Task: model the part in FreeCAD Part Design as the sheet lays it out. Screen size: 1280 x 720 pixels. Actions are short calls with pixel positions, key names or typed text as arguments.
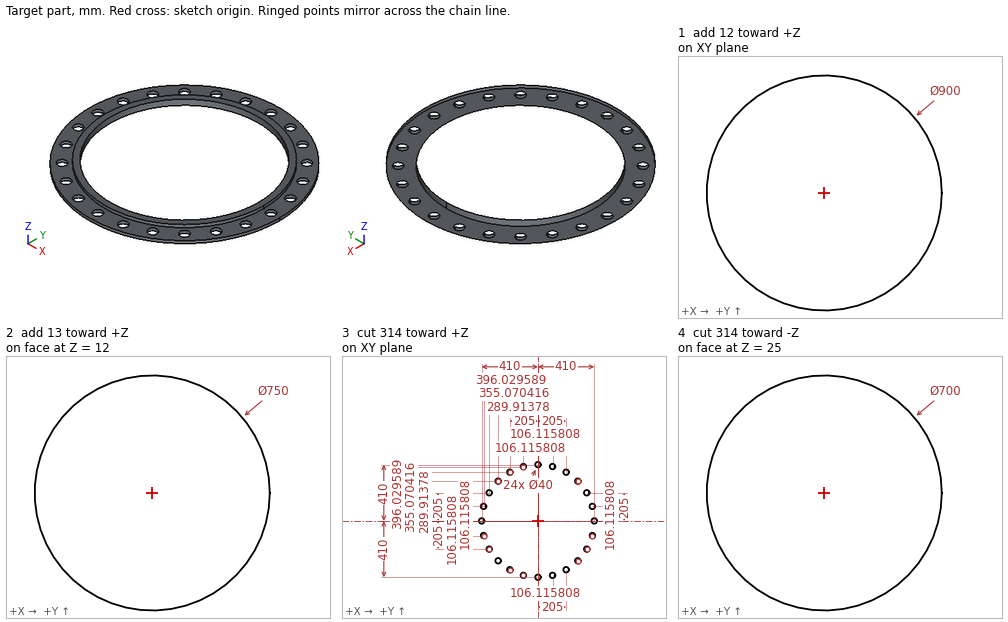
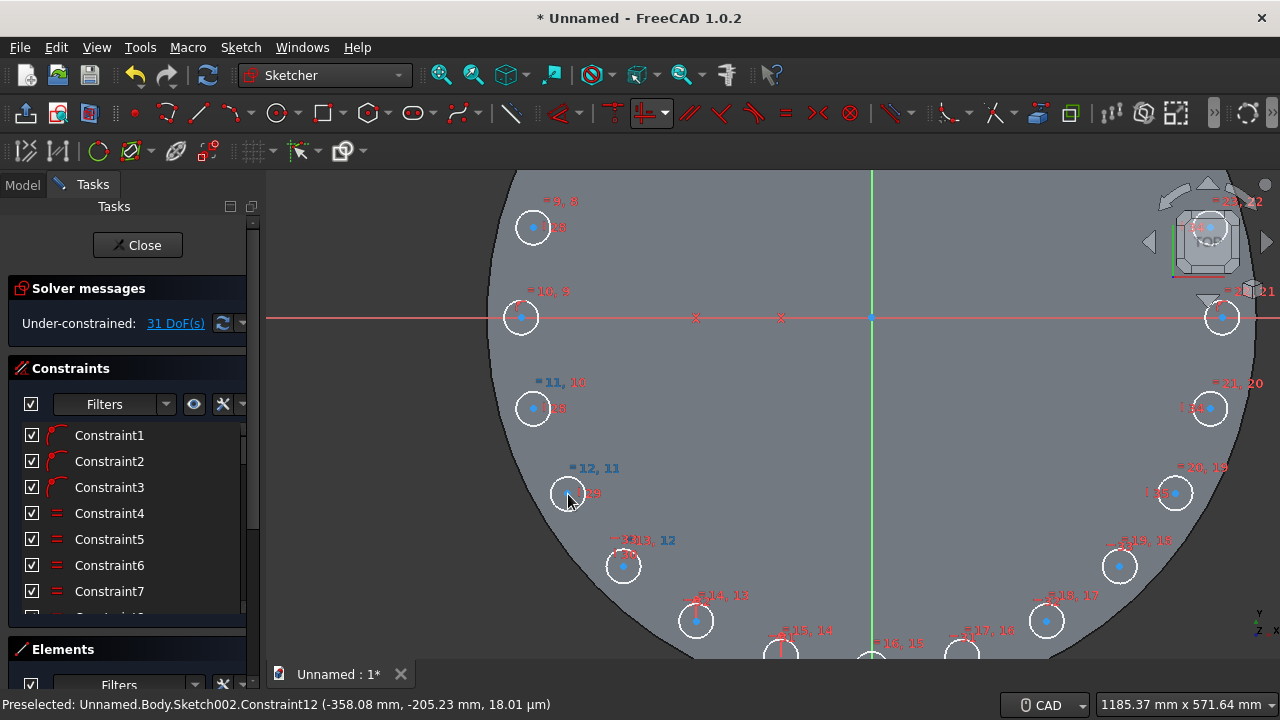
click(568, 494)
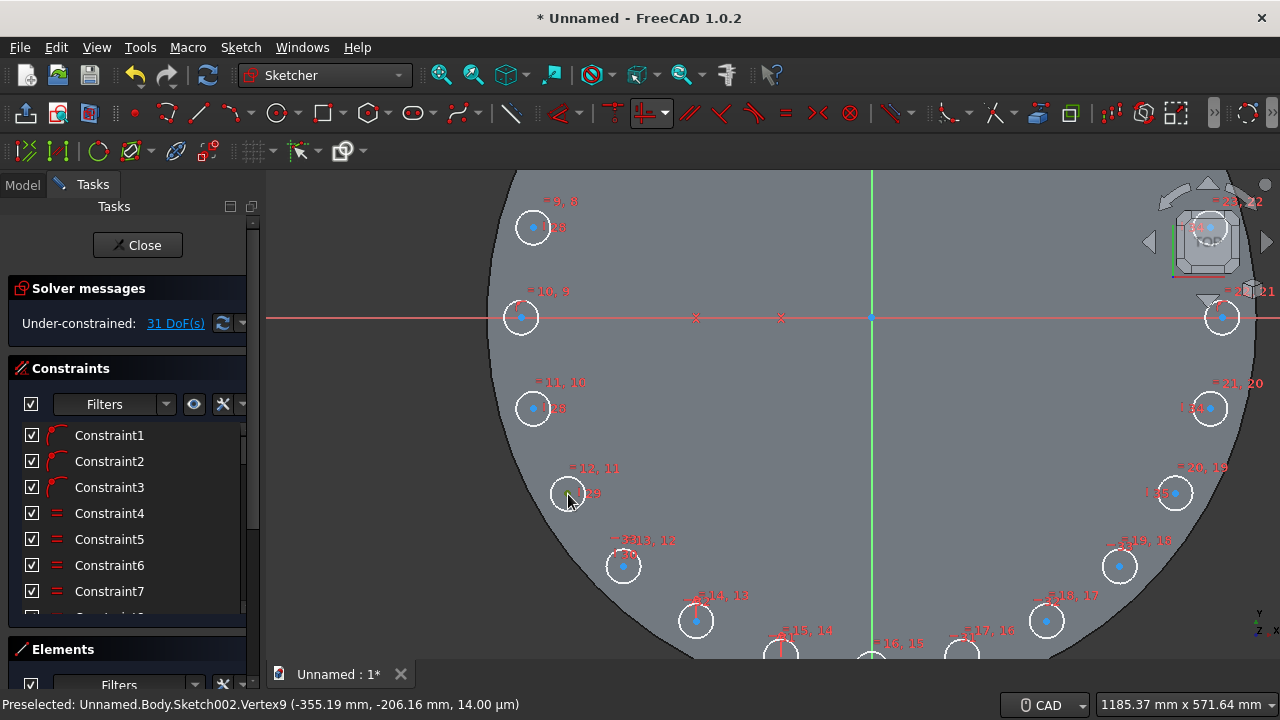
scroll(568, 494, down, 4)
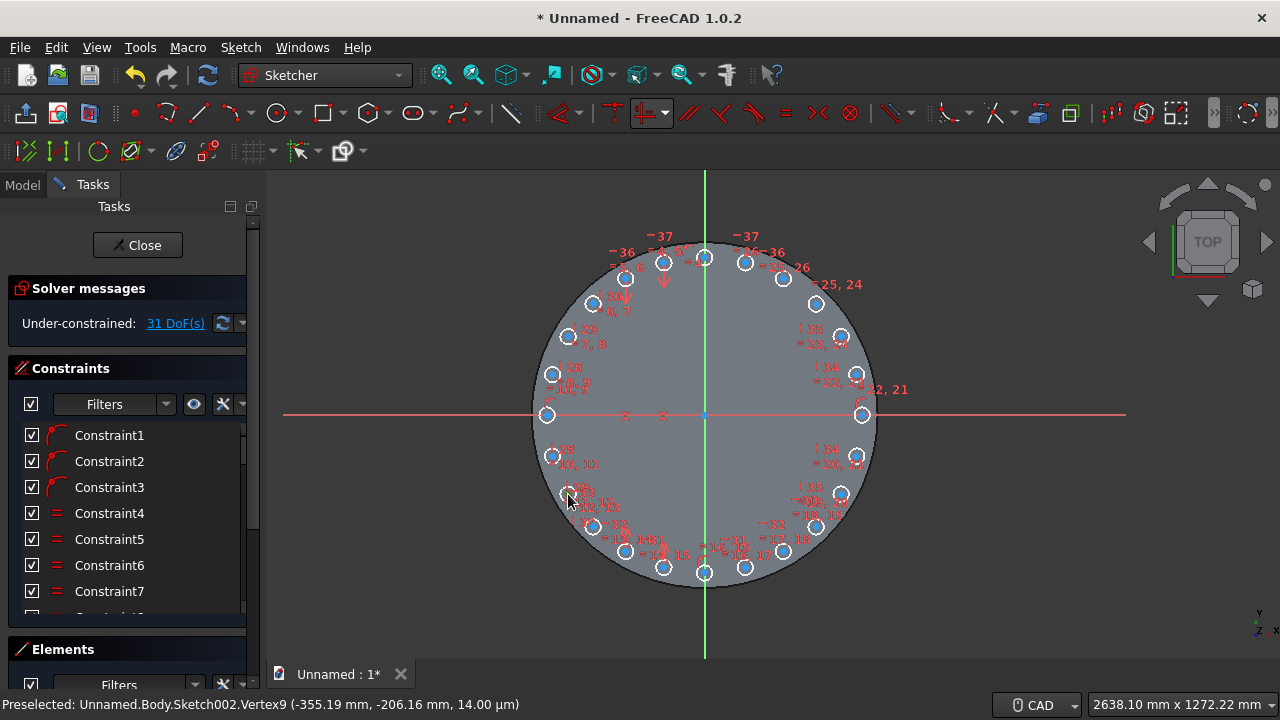
click(843, 496)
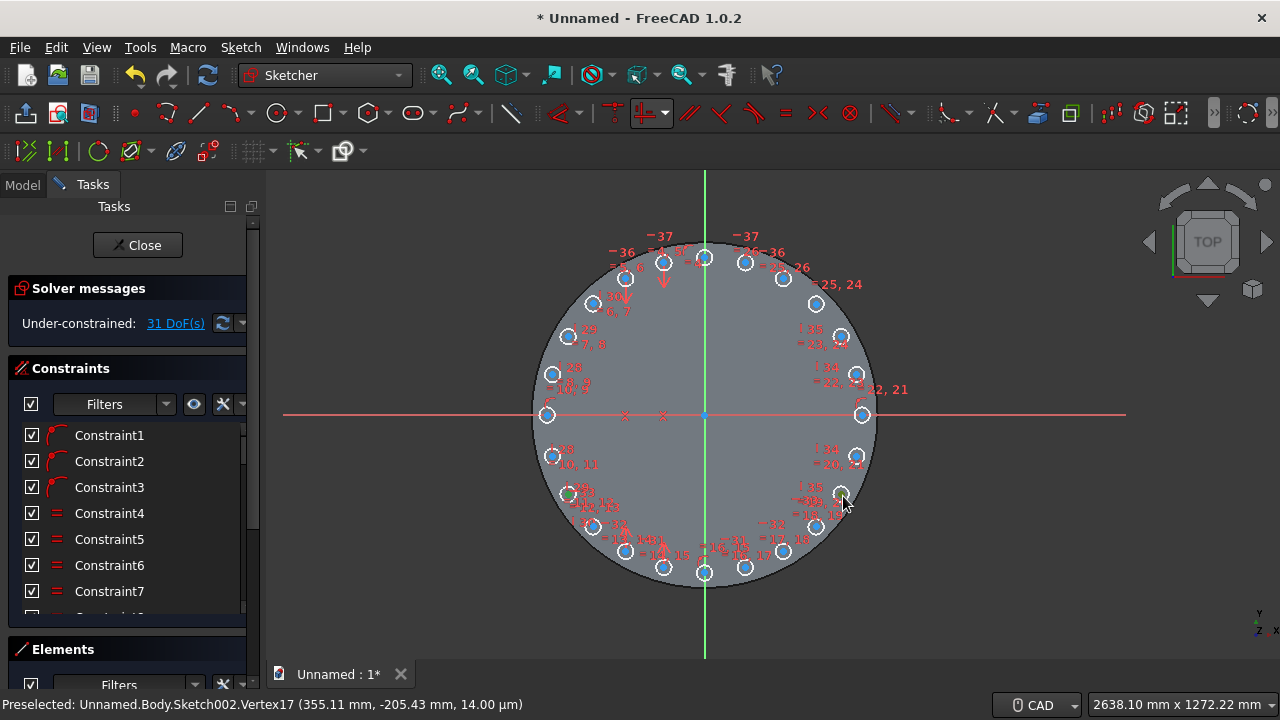
click(705, 507)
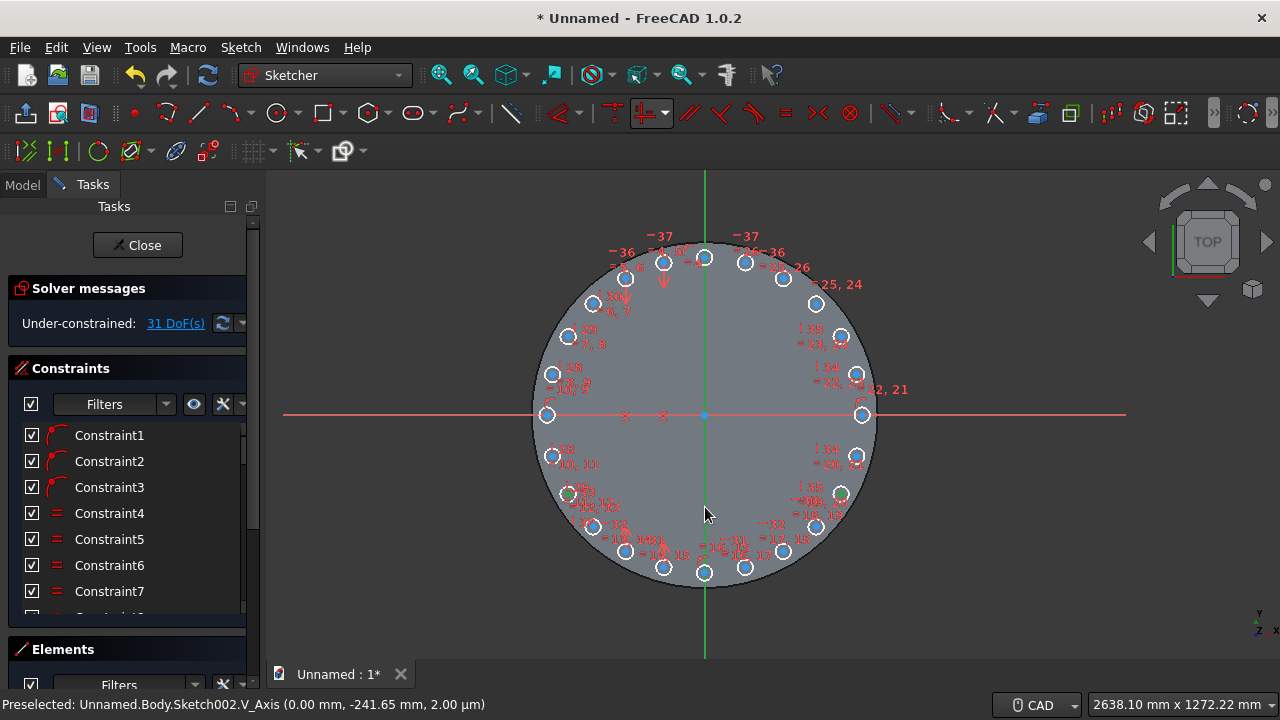
click(818, 114)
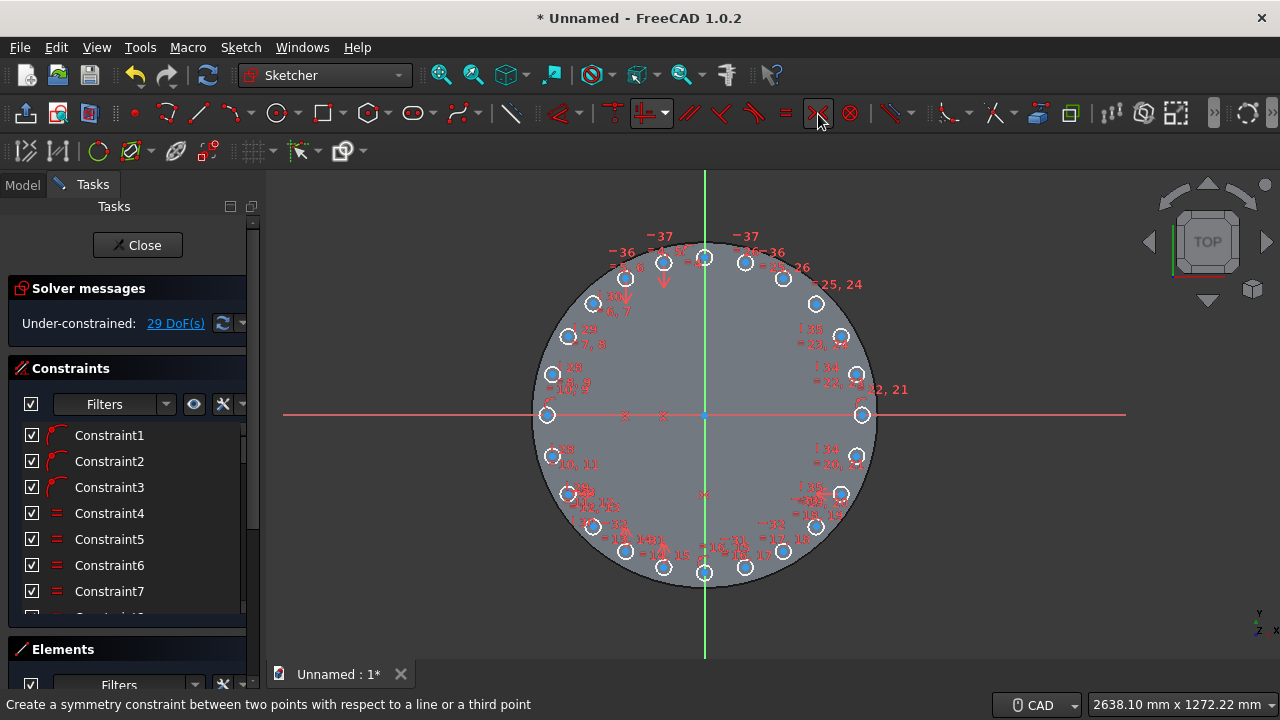
scroll(553, 456, up, 4)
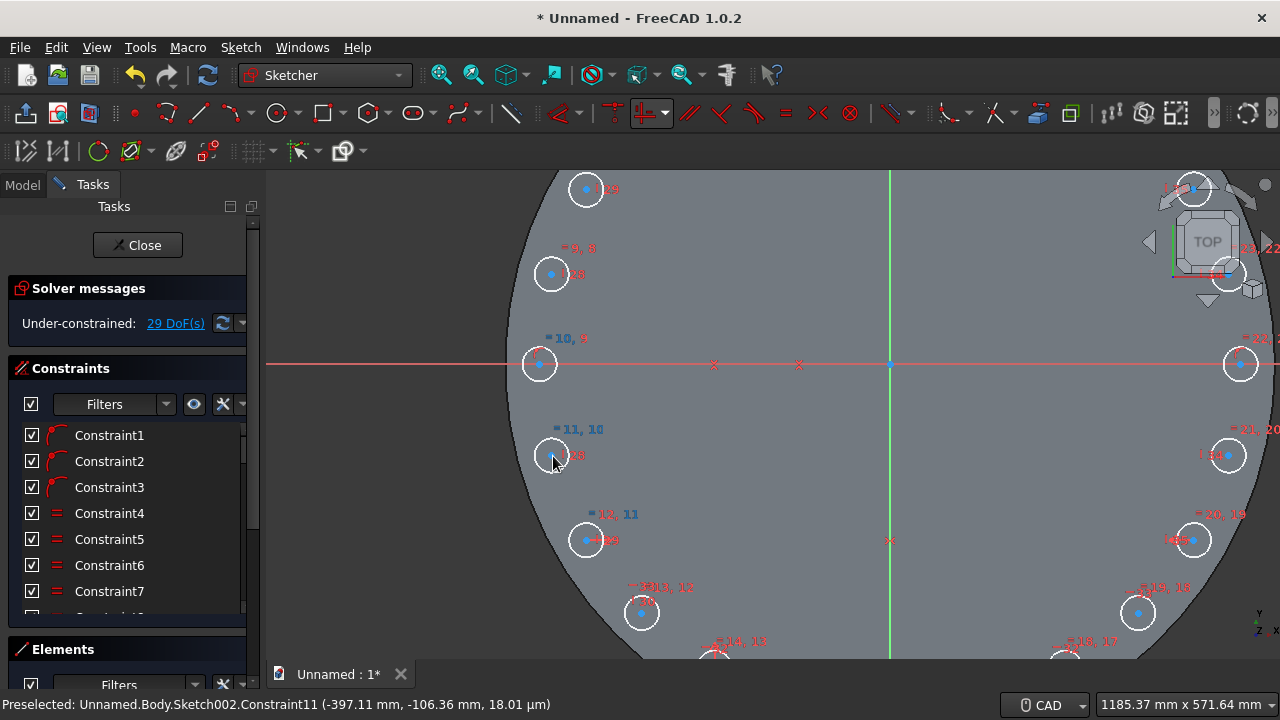
click(552, 456)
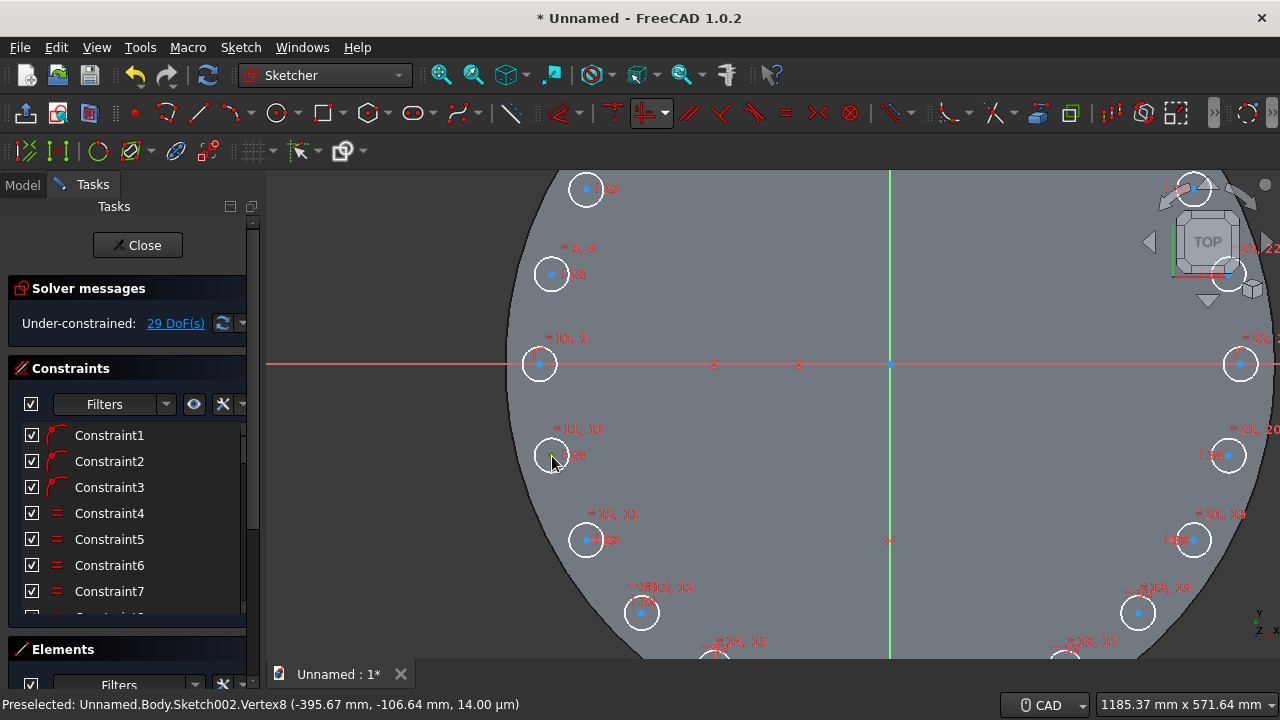
scroll(553, 455, down, 4)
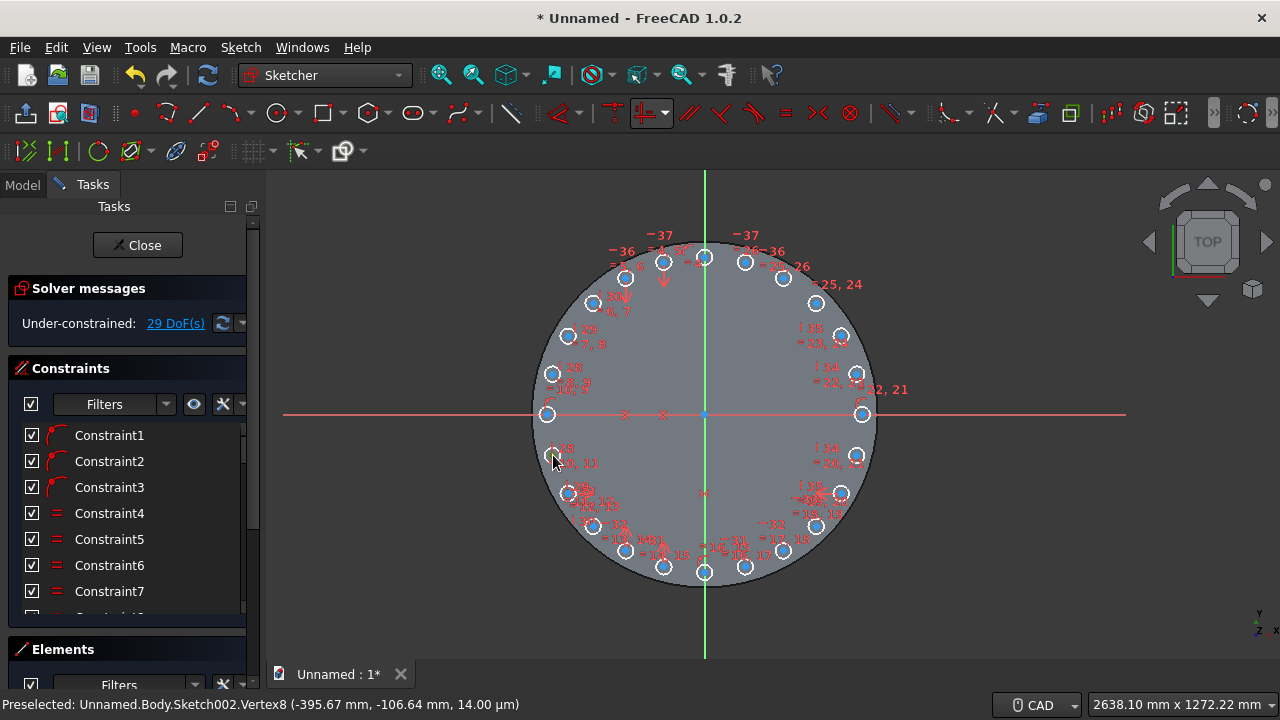
click(857, 456)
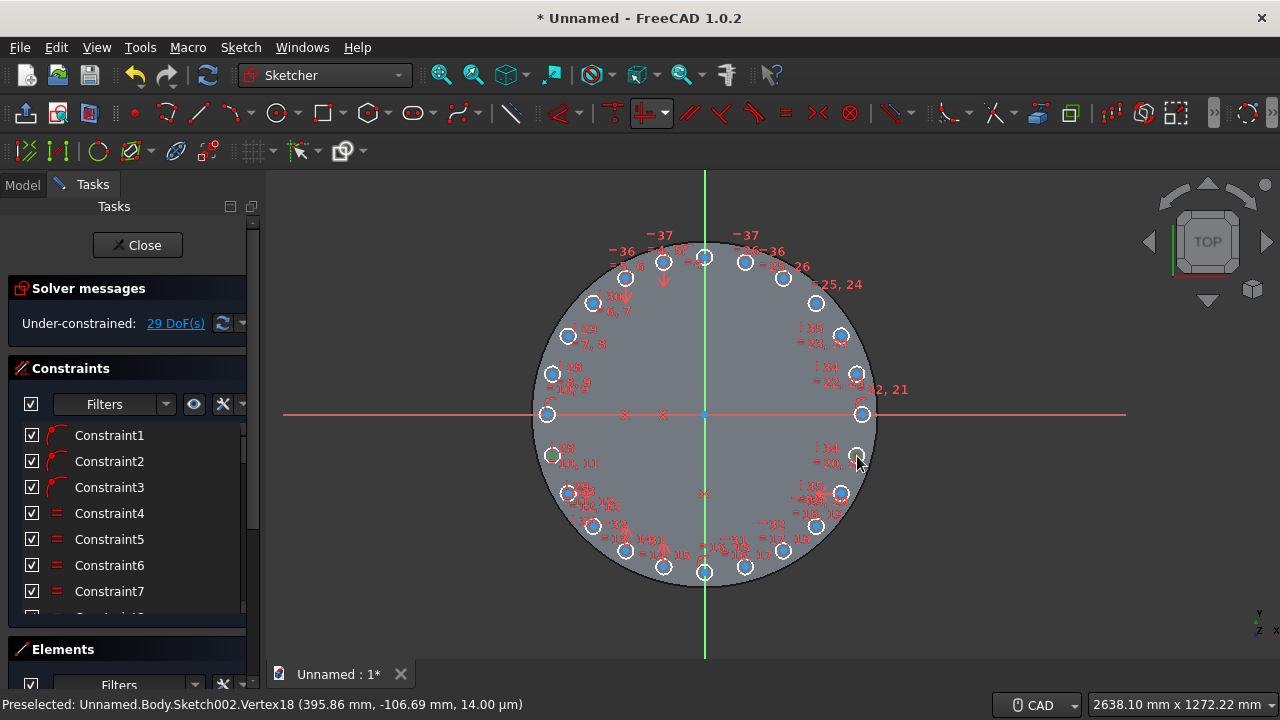
click(705, 507)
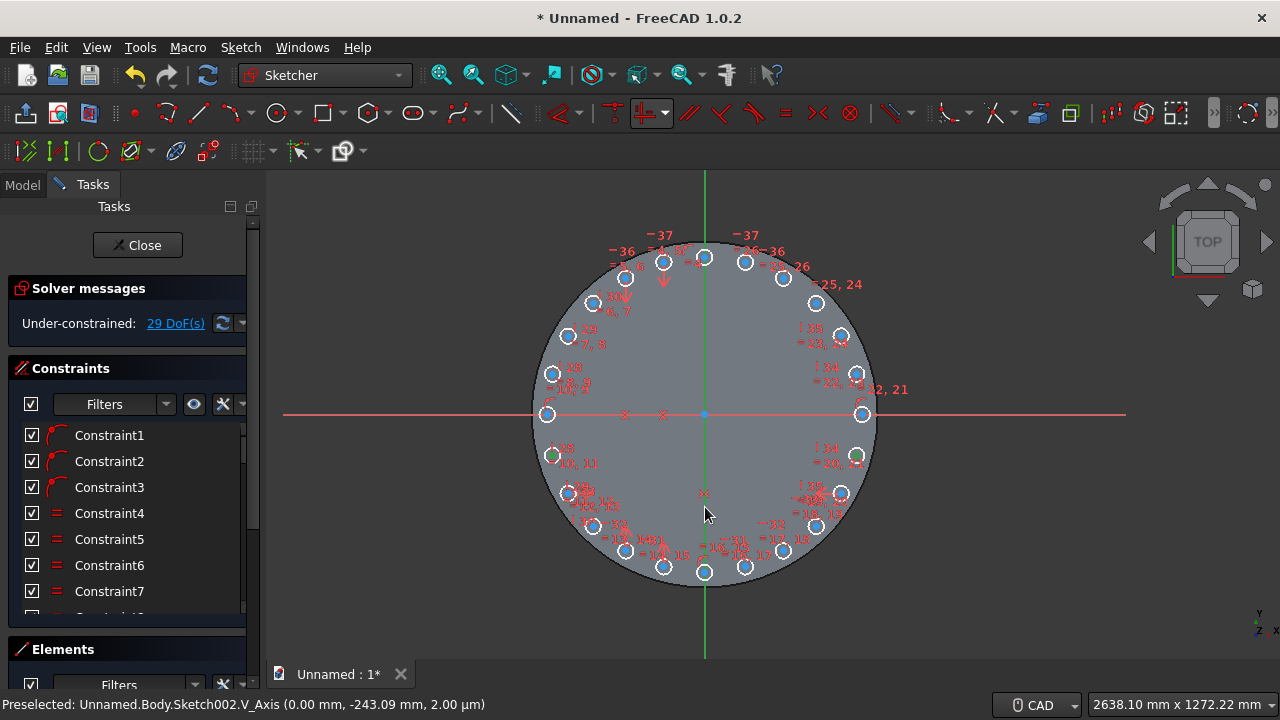
click(818, 114)